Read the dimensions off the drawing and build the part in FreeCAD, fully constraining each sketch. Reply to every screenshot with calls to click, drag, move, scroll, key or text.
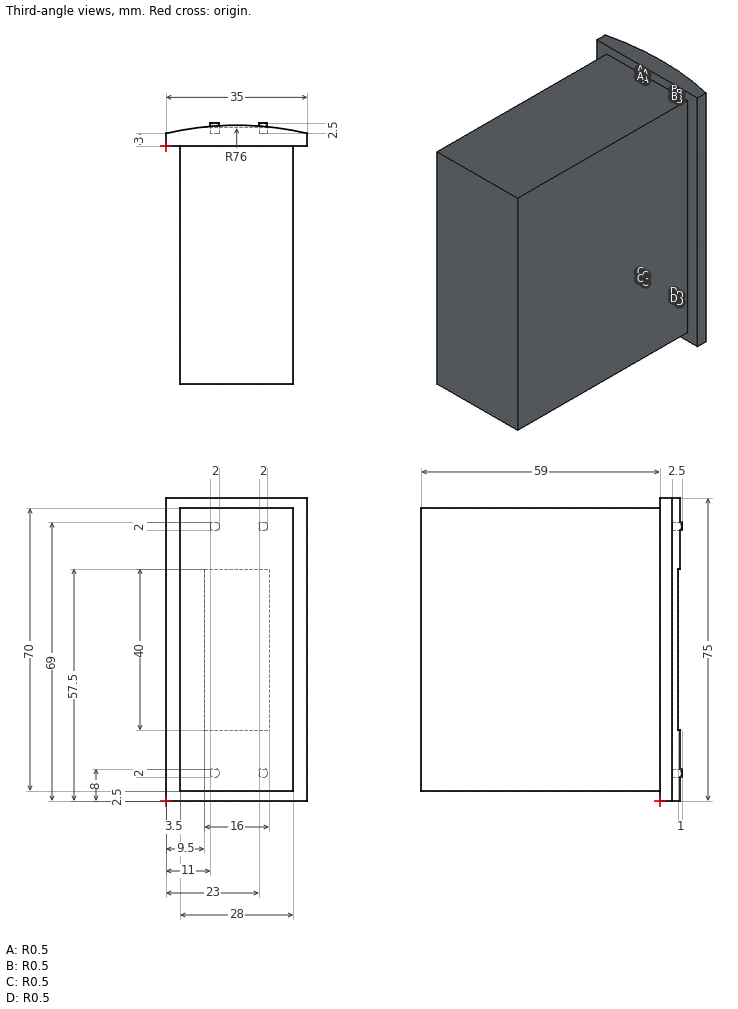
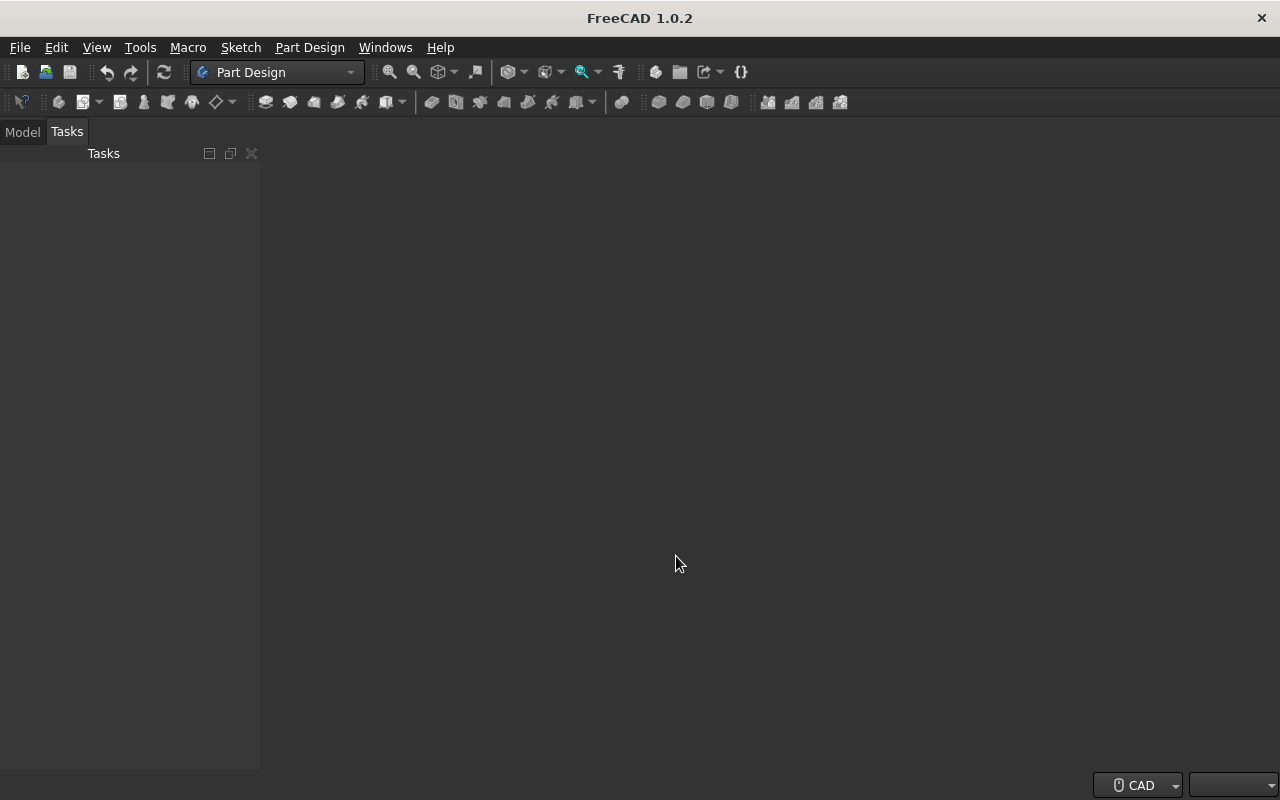
key(ctrl+n)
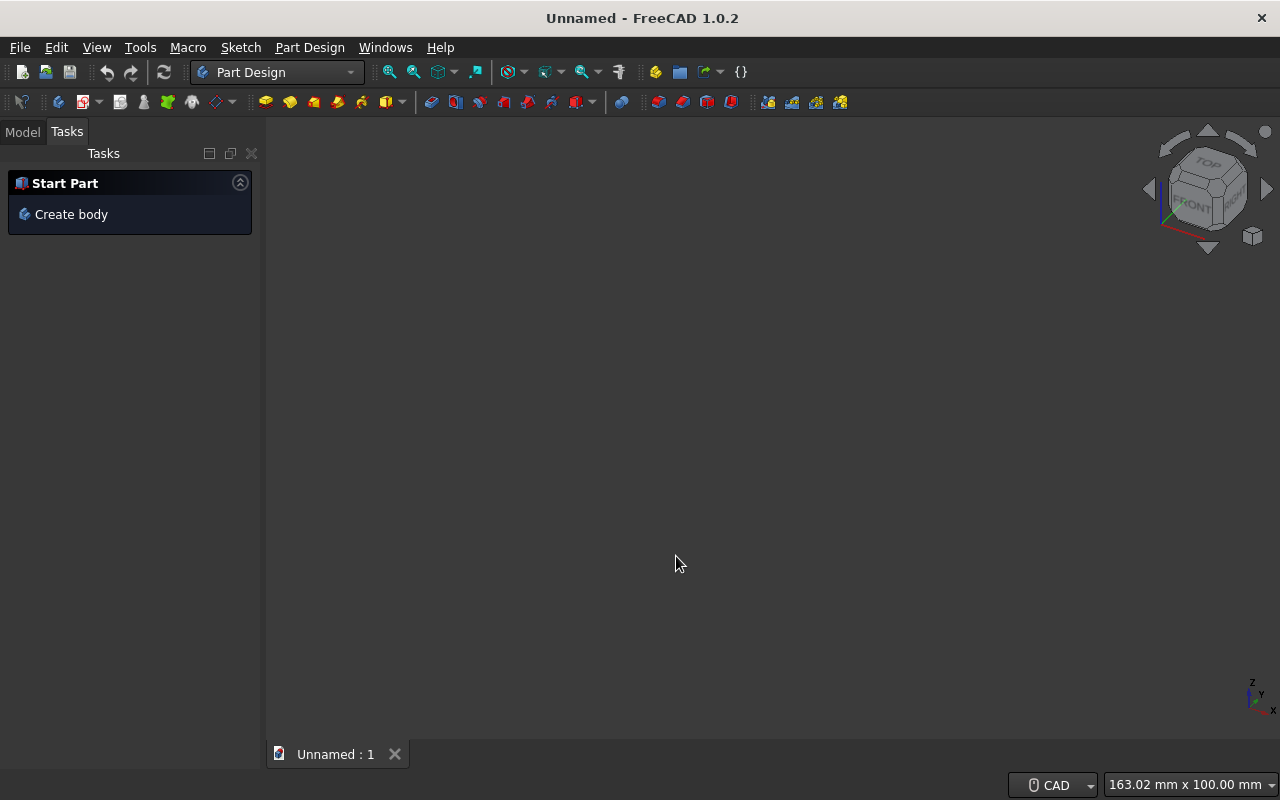
click(84, 102)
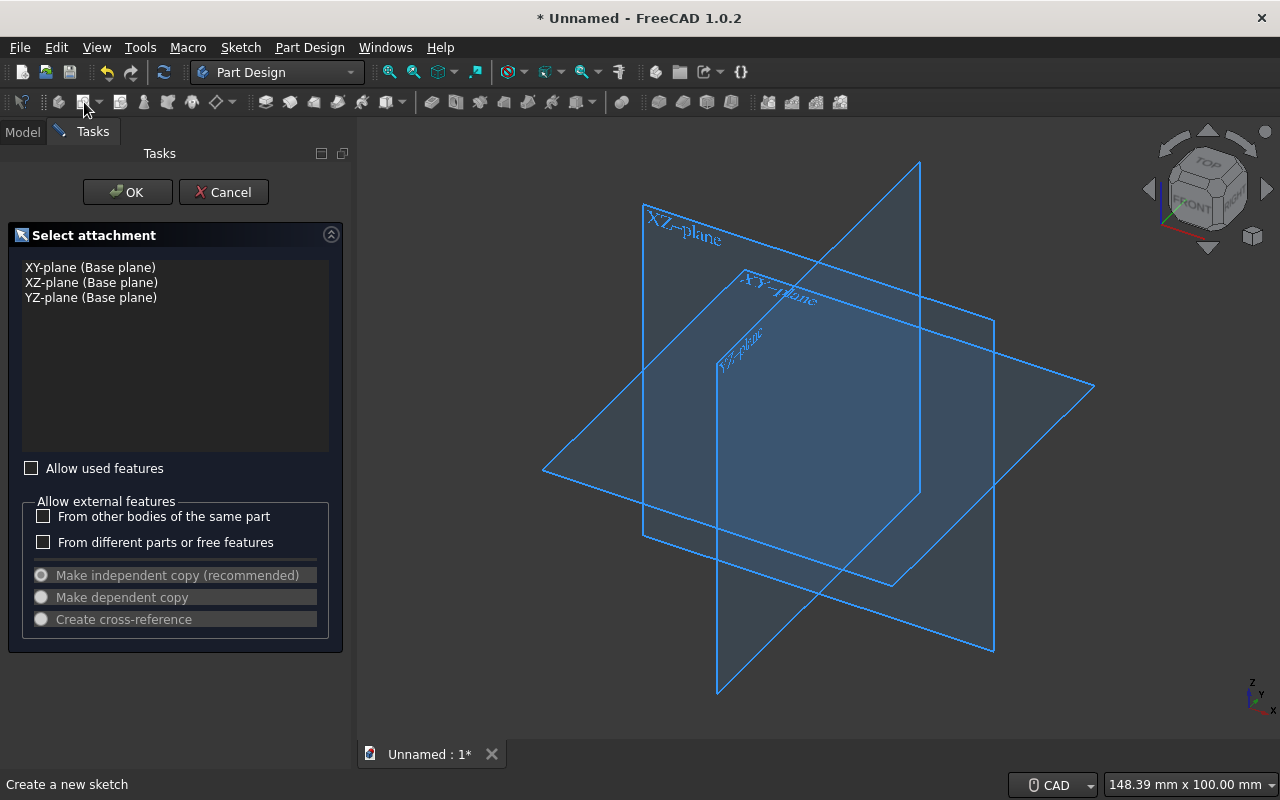
click(82, 268)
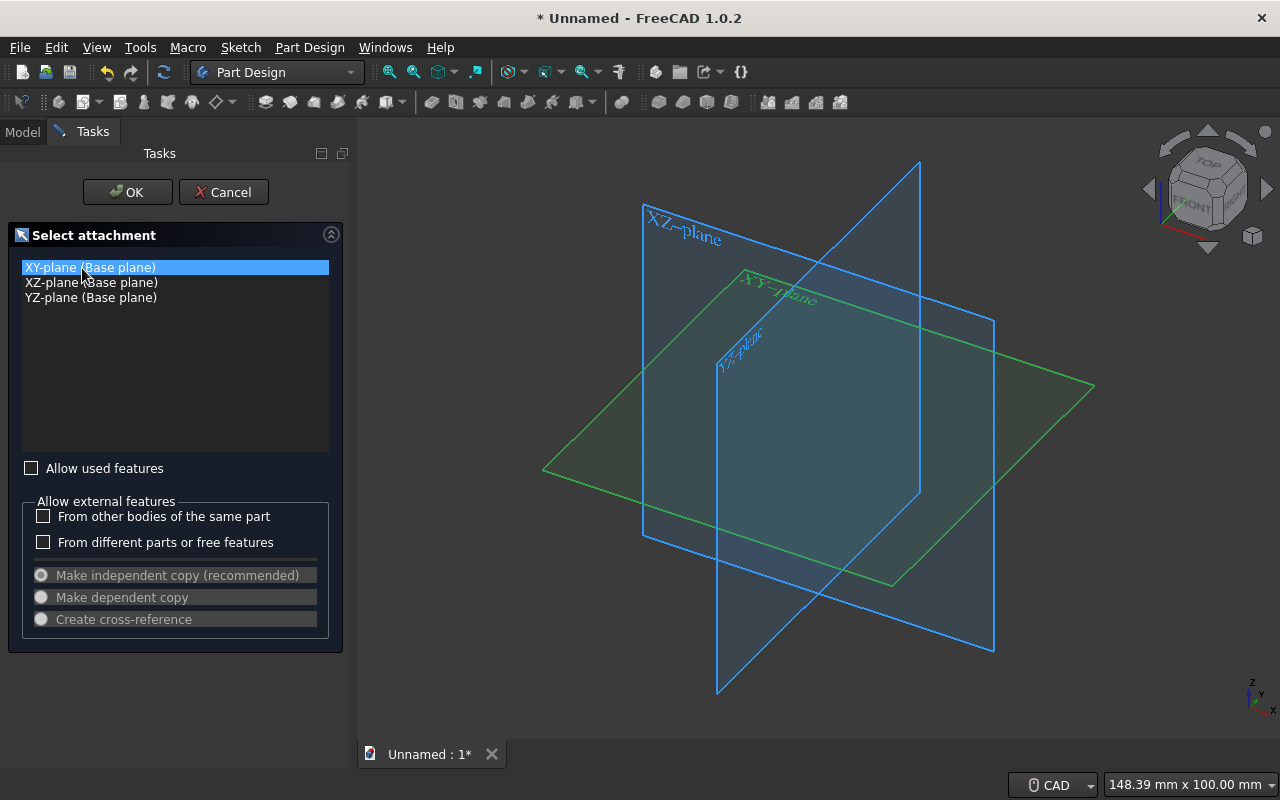
click(128, 192)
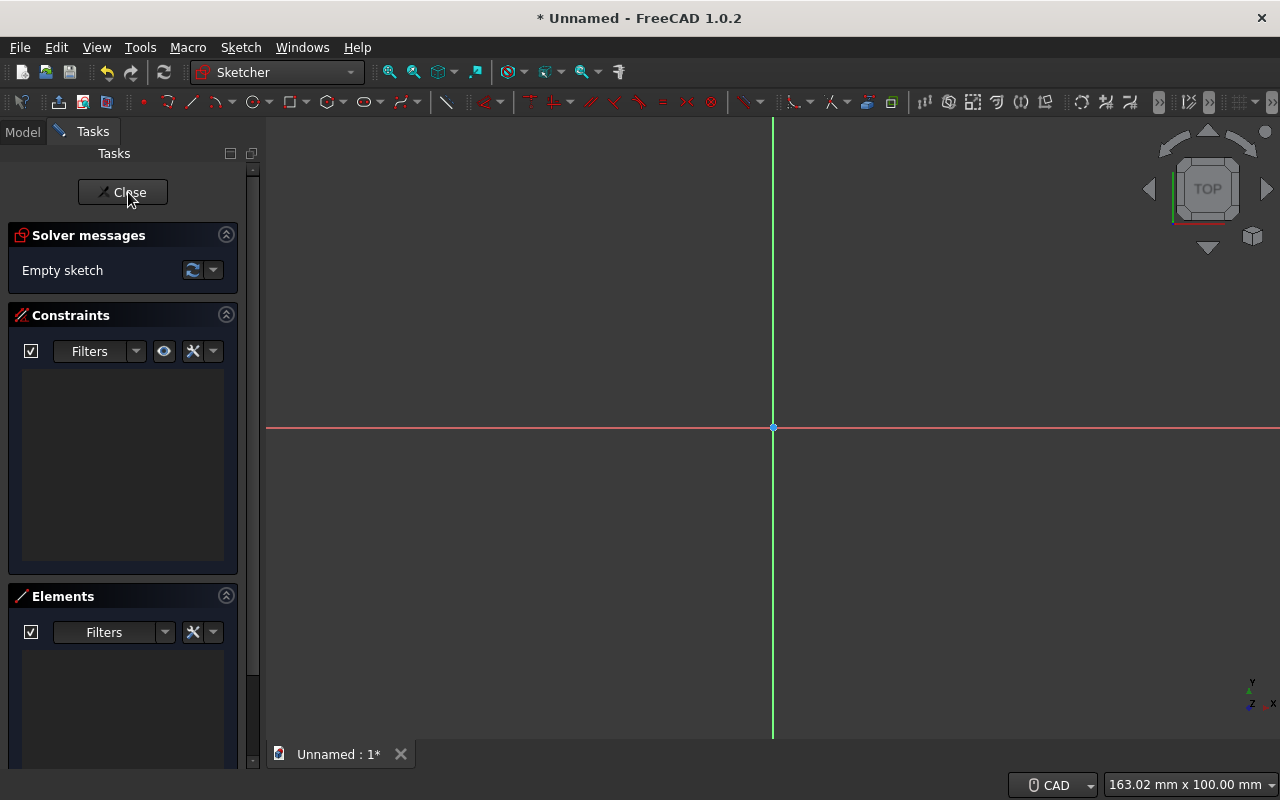
scroll(985, 403, up, 5)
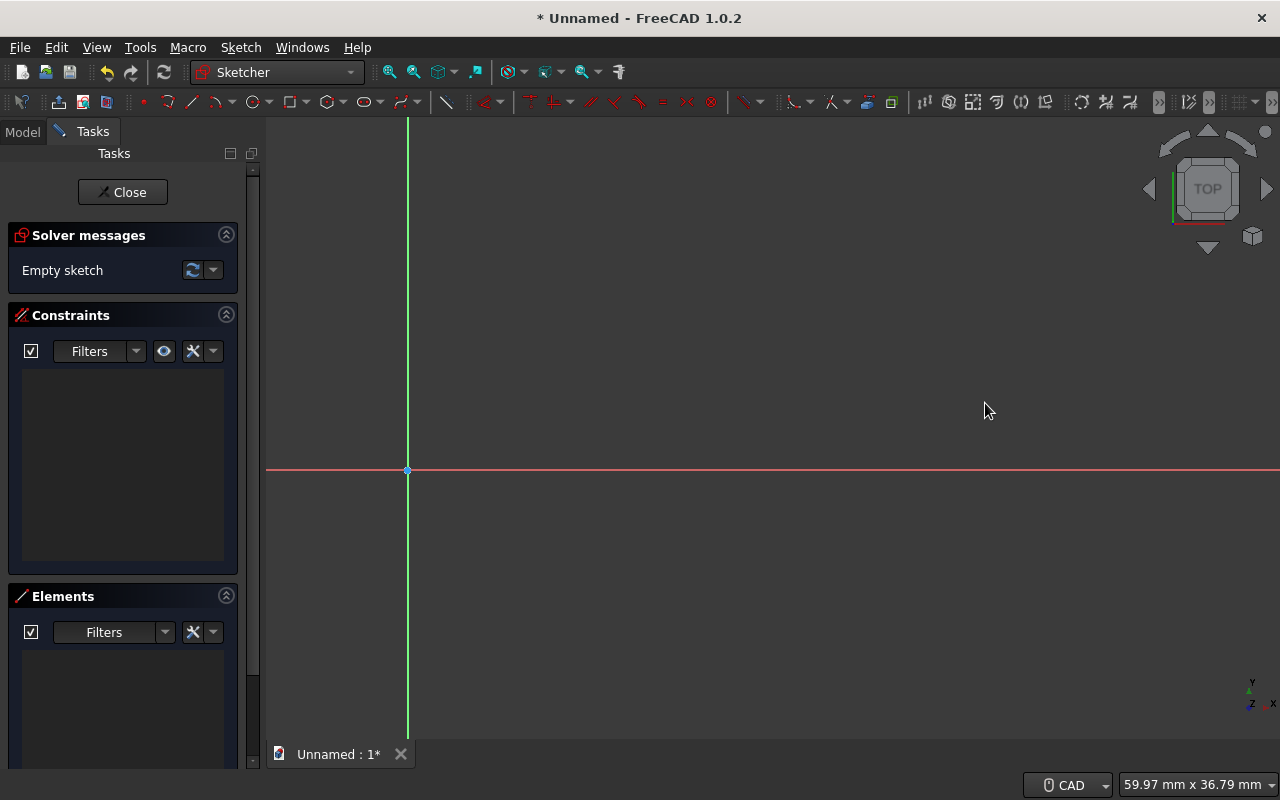
key(g)
key(m)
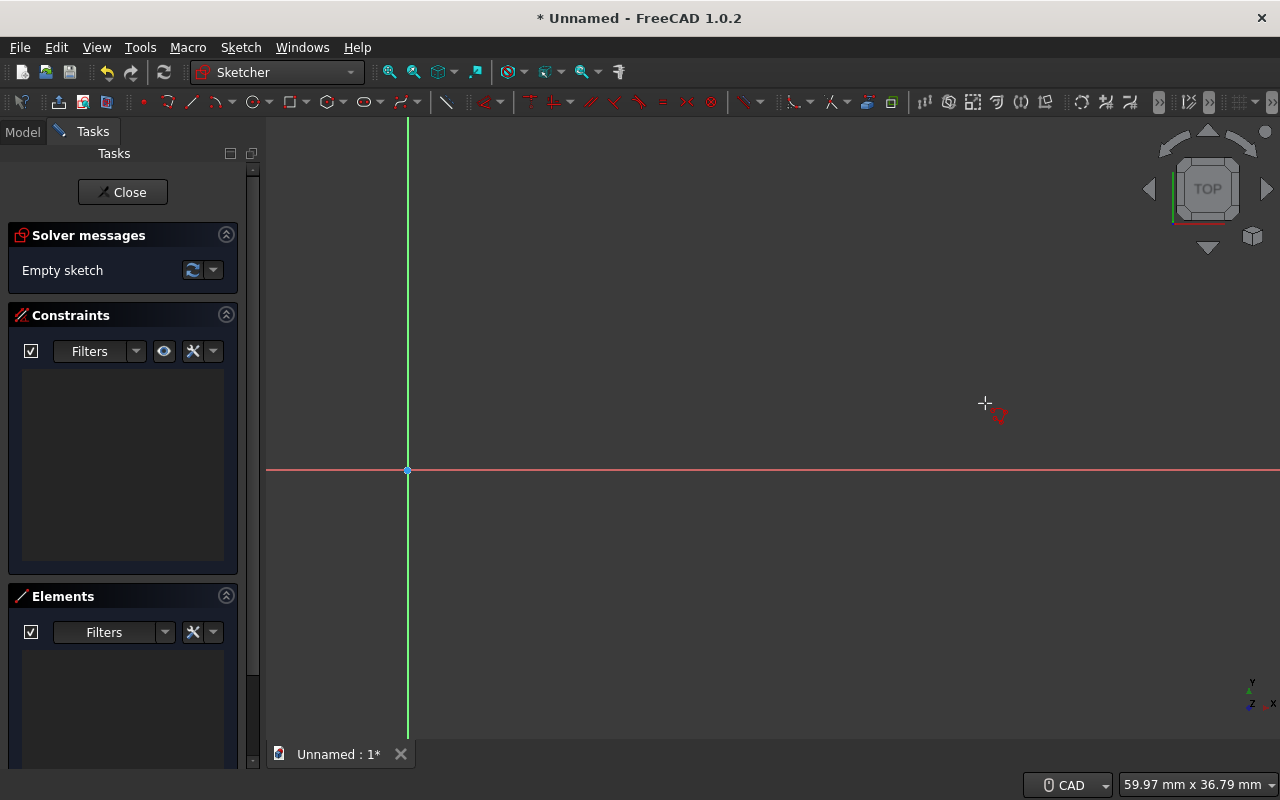
click(408, 419)
click(408, 470)
click(999, 461)
click(999, 419)
right_click(999, 419)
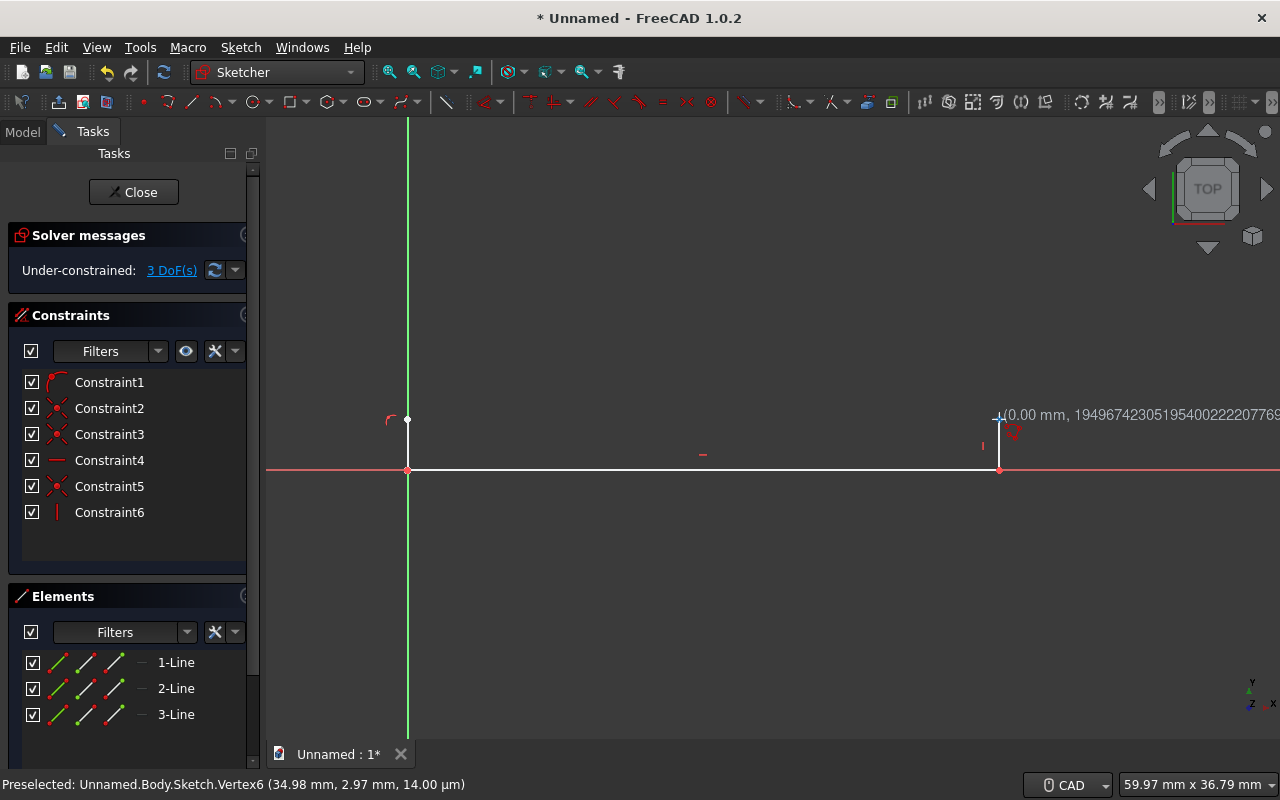
key(g)
key(3)
key(a)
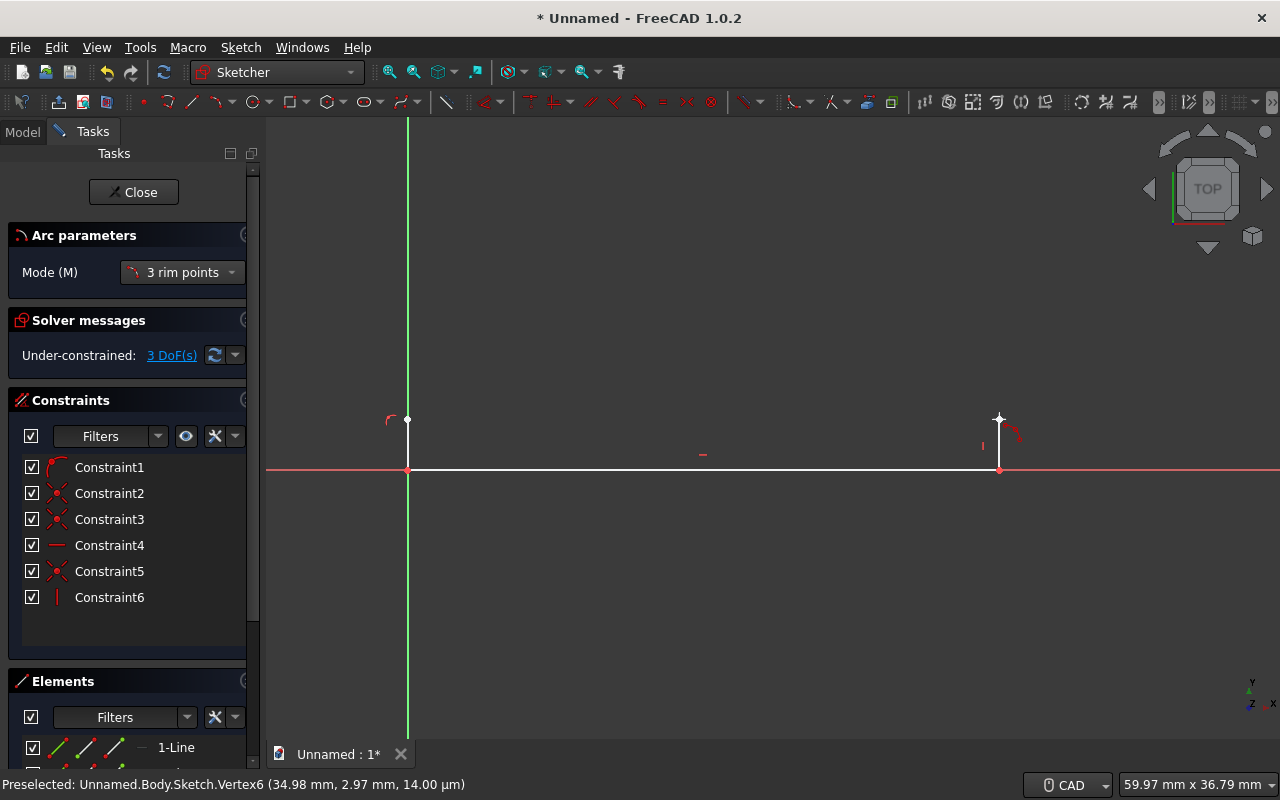
click(999, 420)
click(408, 420)
click(703, 385)
key(Escape)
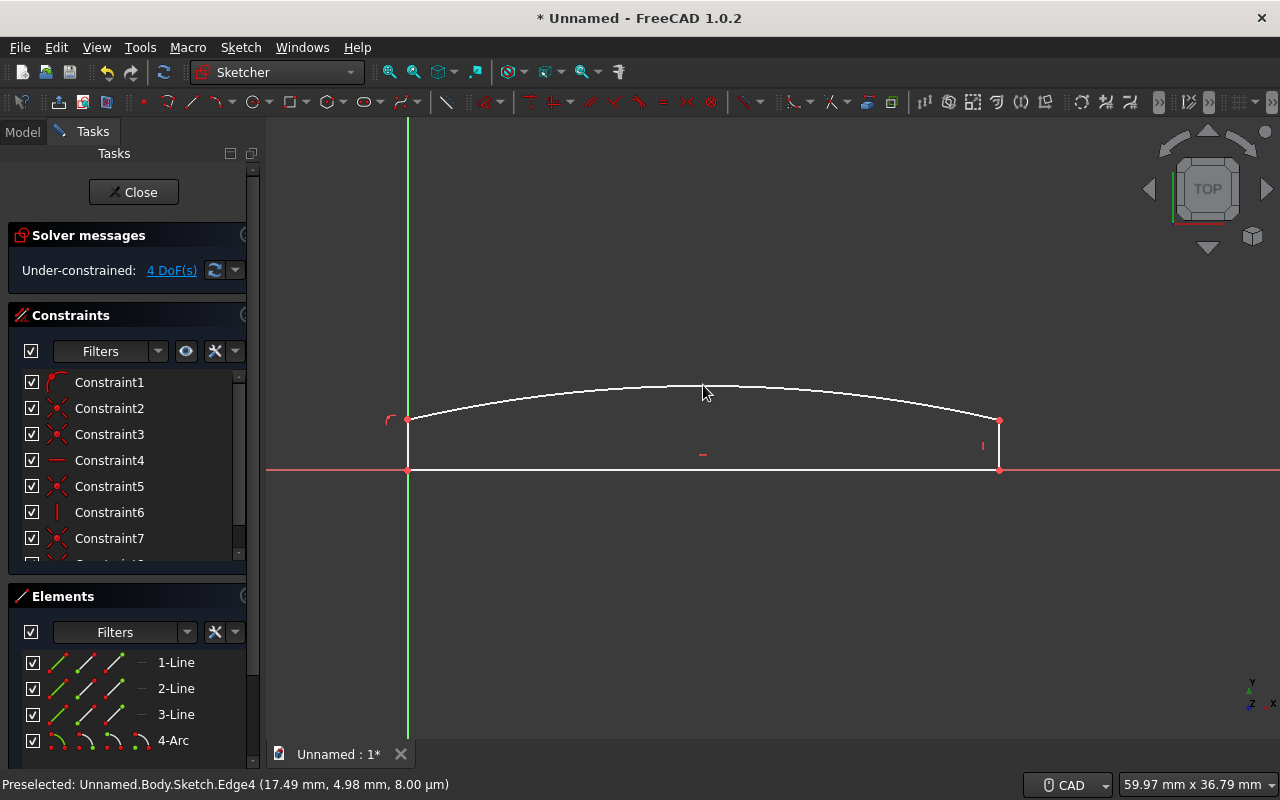
key(d)